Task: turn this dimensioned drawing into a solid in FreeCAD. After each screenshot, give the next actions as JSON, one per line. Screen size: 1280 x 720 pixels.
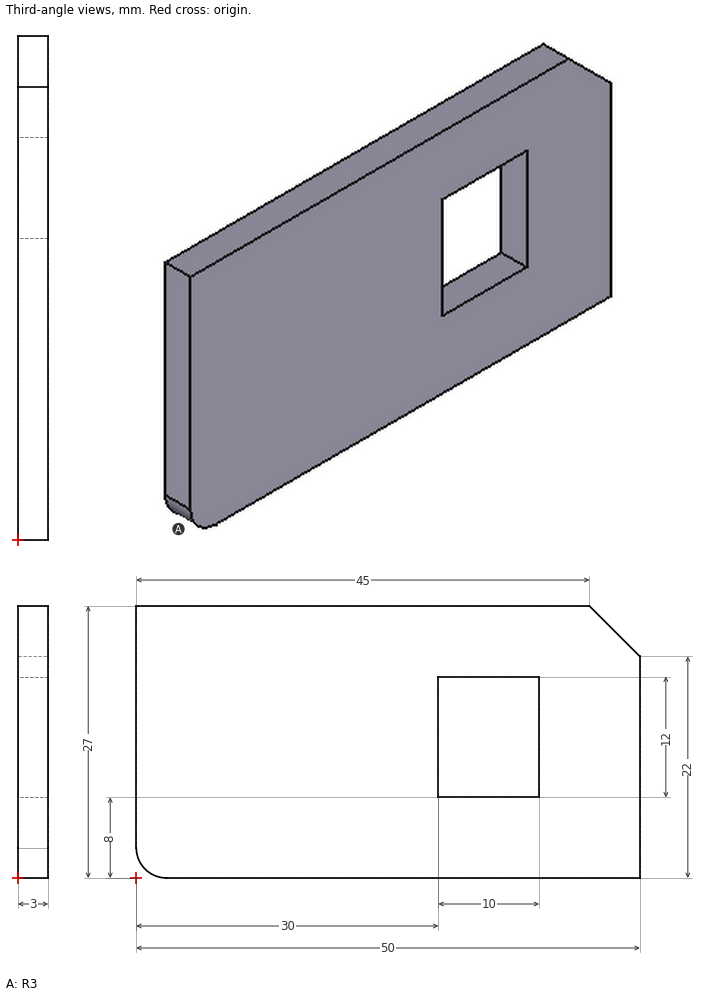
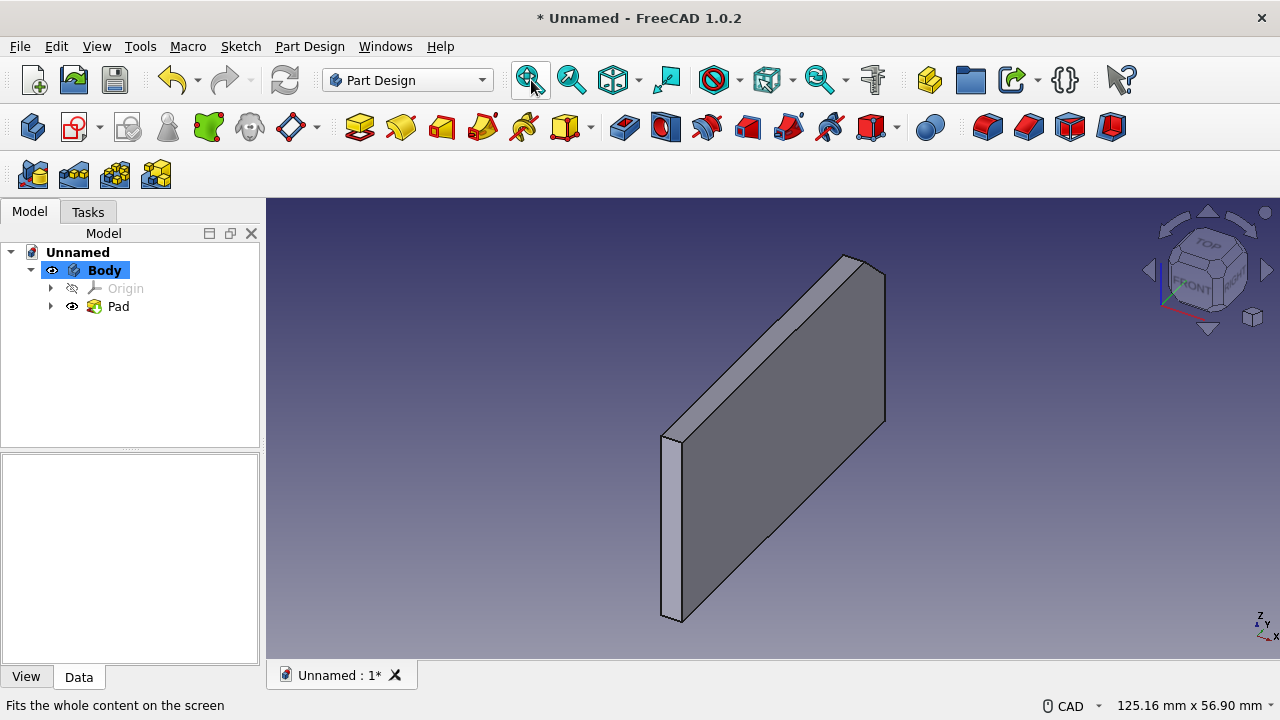
{"action": "key", "text": "0"}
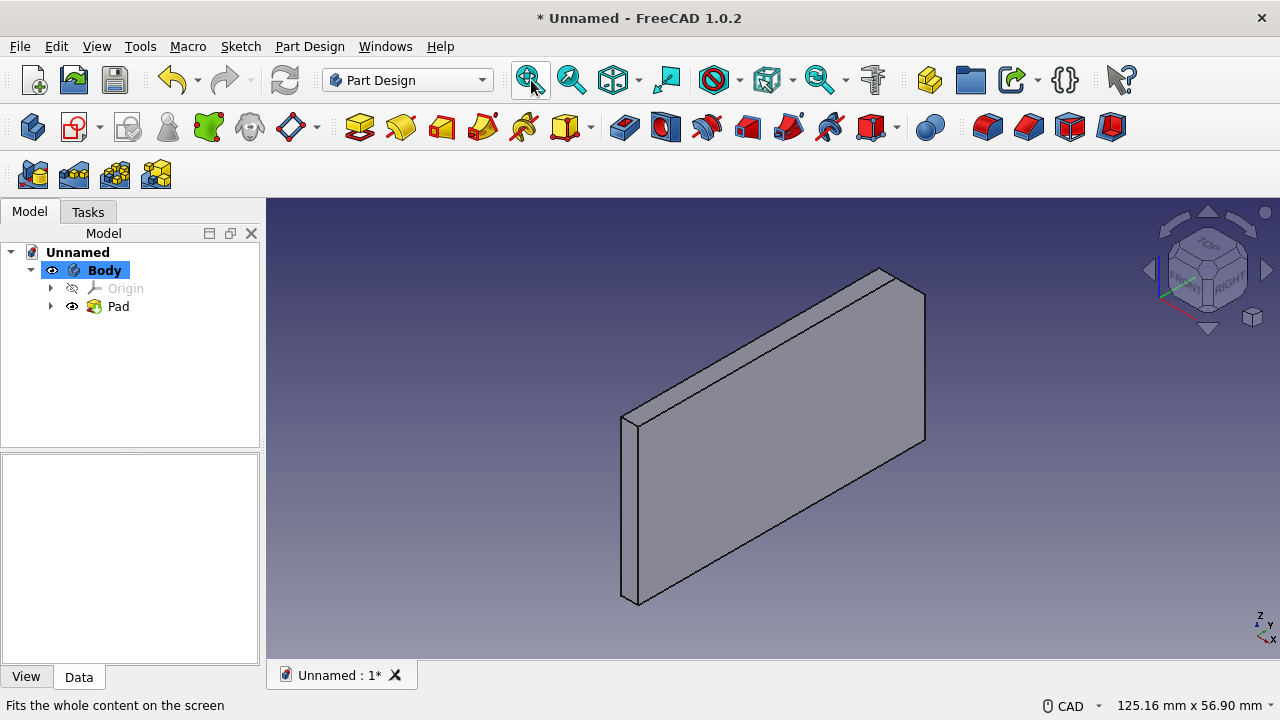
{"action": "key", "text": "2"}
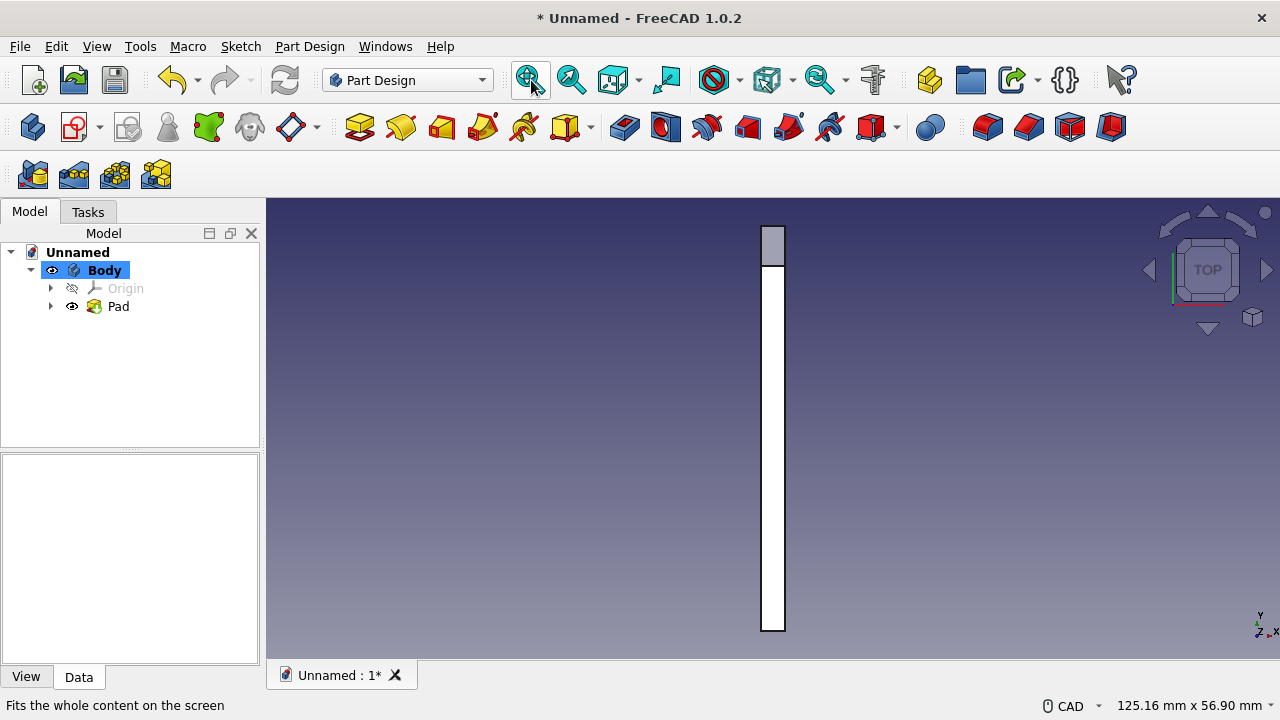
{"action": "key", "text": "1"}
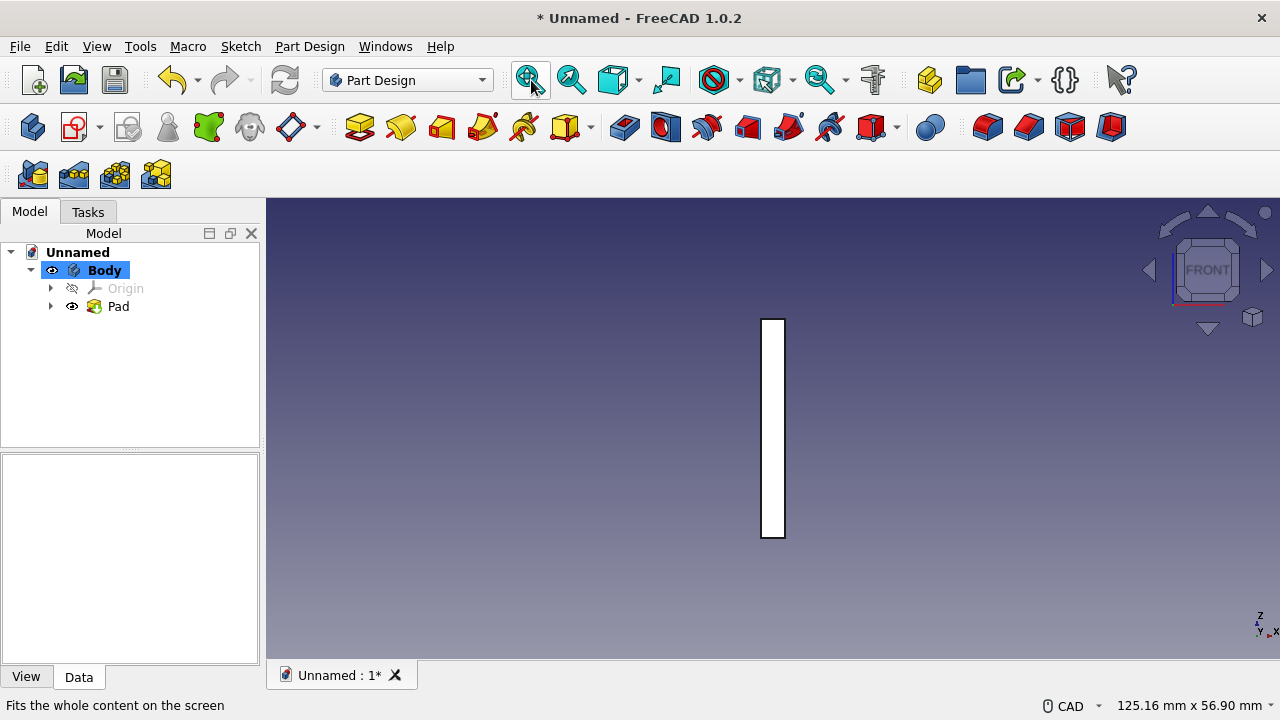
{"action": "key", "text": "3"}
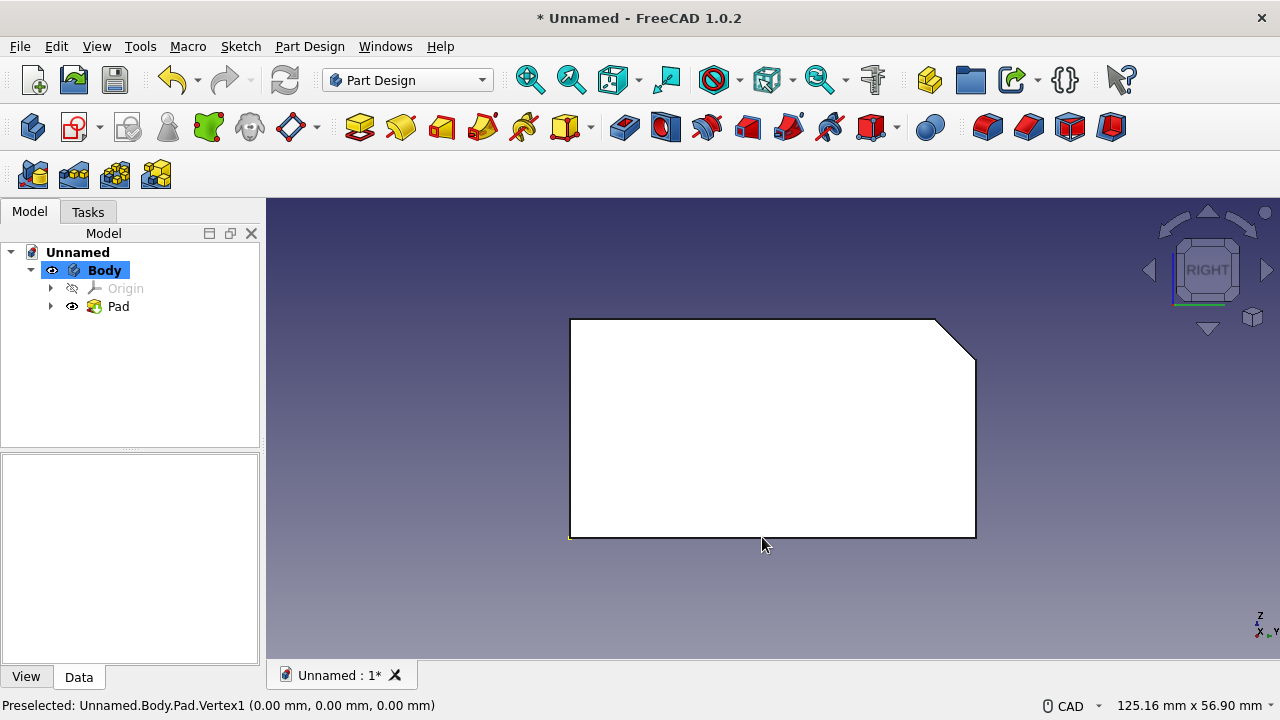
{"action": "key", "text": "5"}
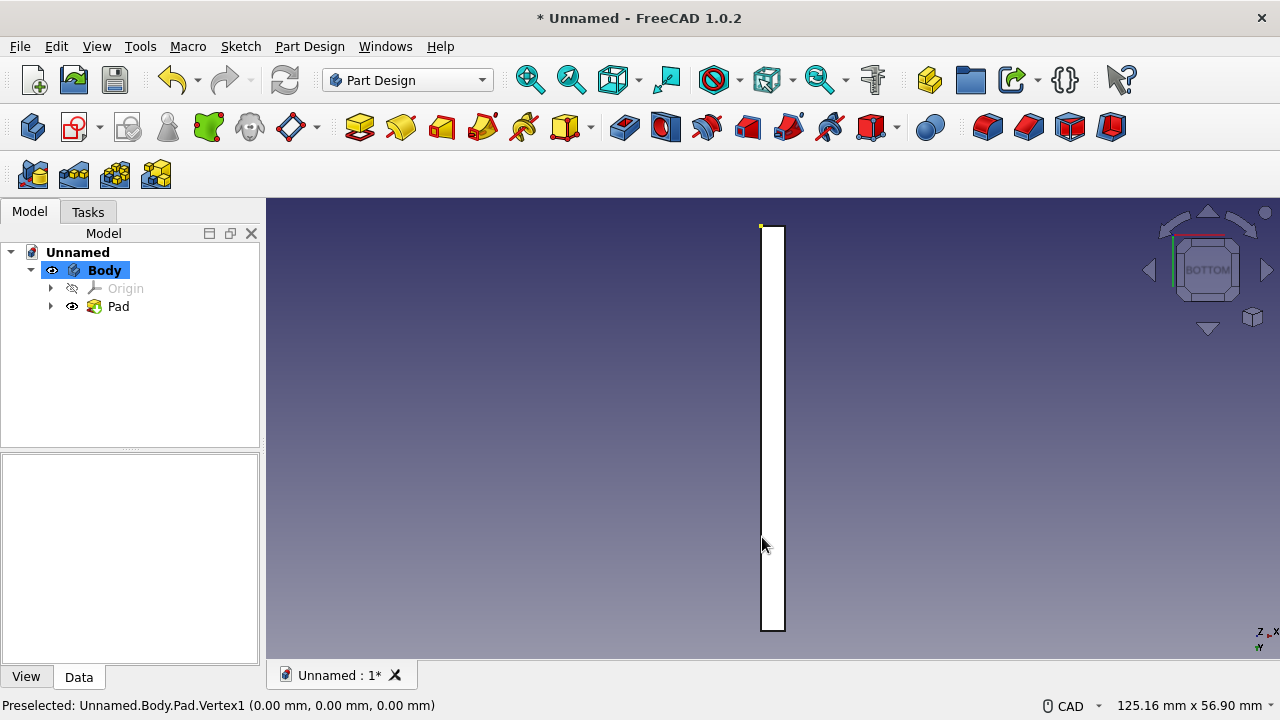
{"action": "key", "text": "4"}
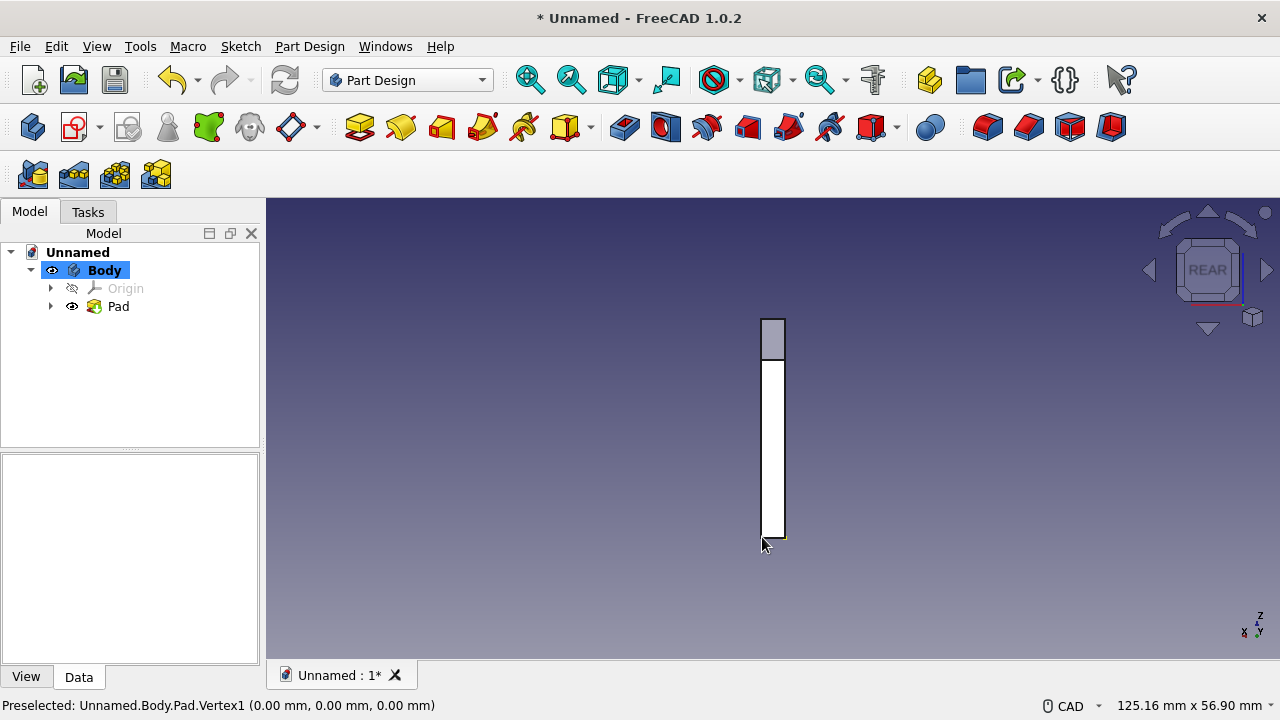
{"action": "key", "text": "6"}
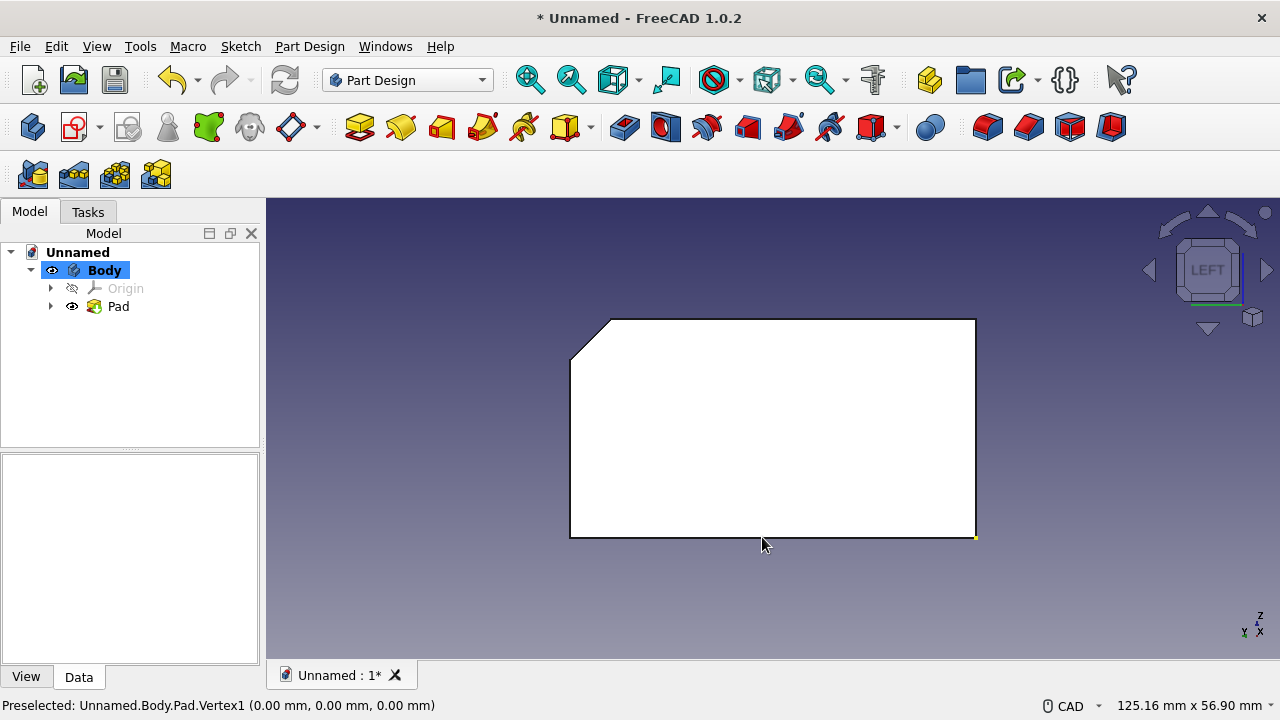
{"action": "key", "text": "v 3"}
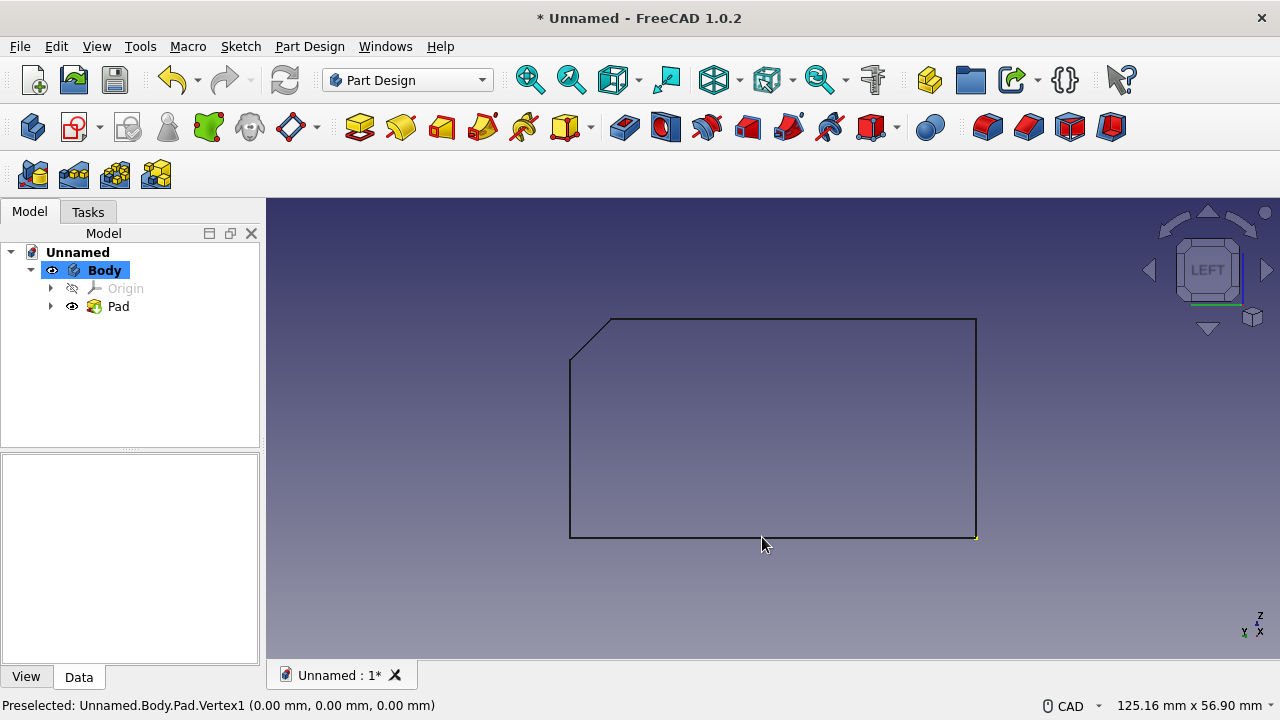
{"action": "key", "text": "0"}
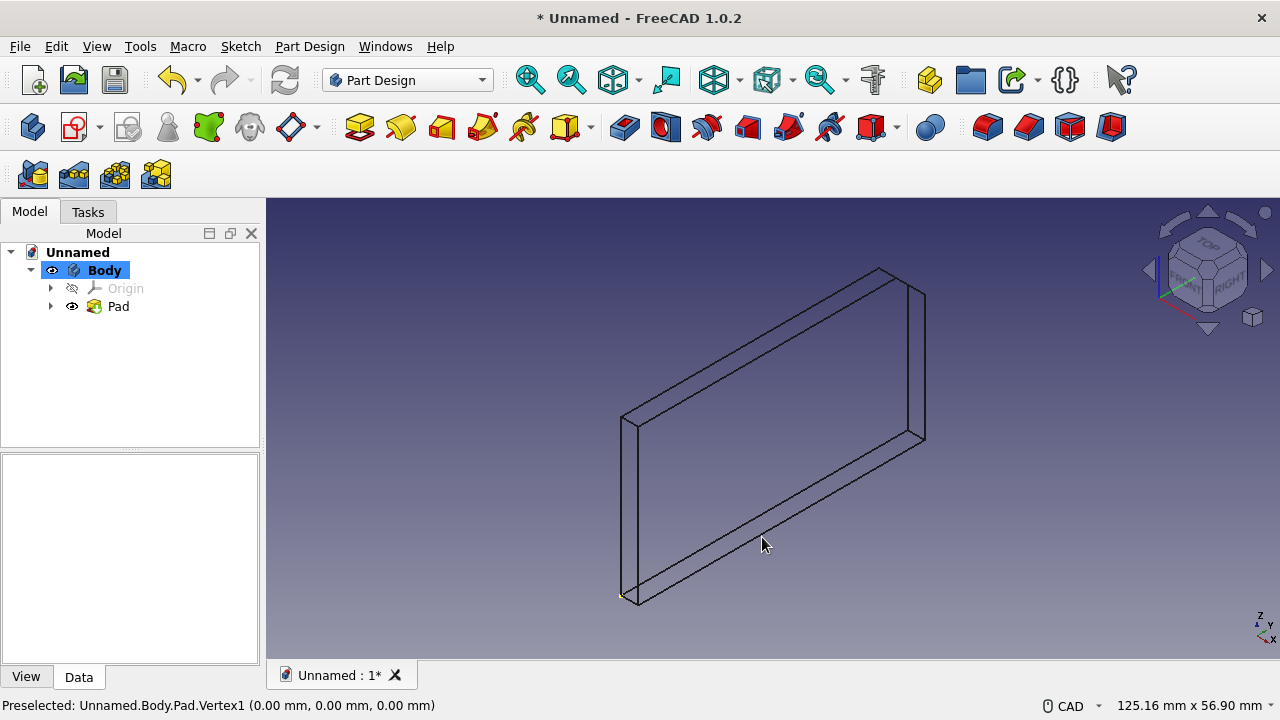
{"action": "left_click", "coordinate": [630, 599]}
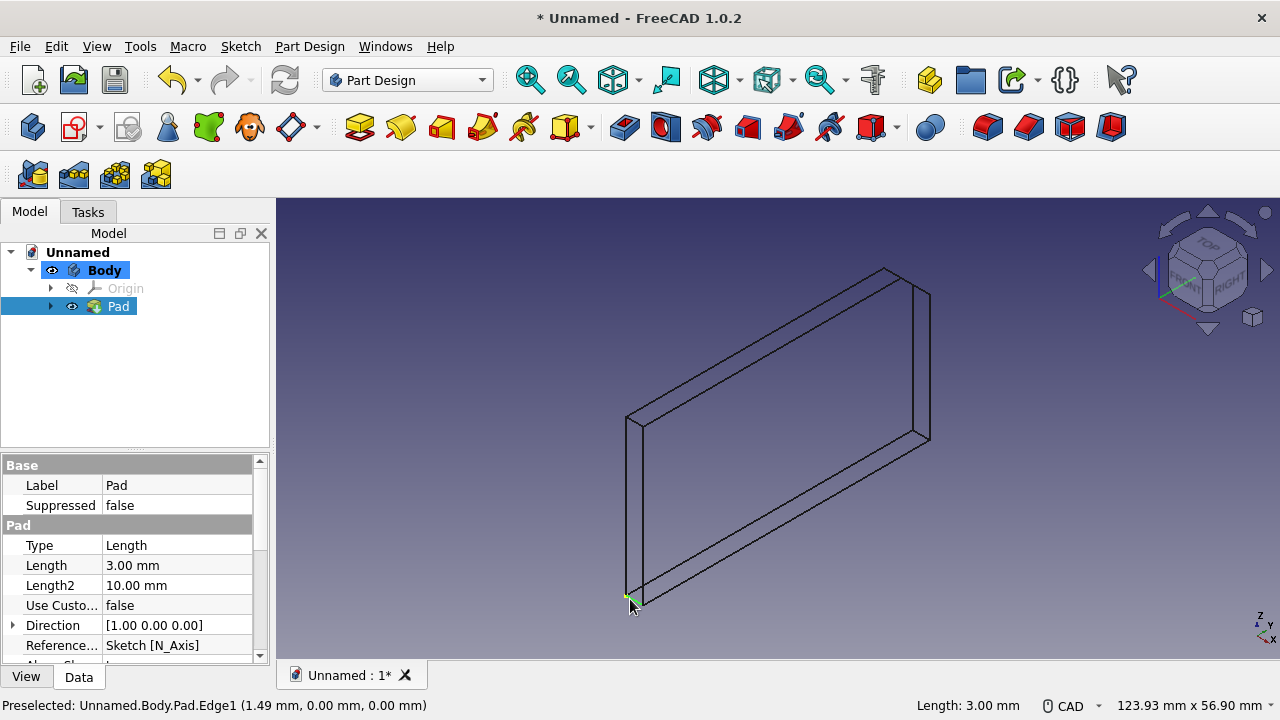
{"action": "key", "text": "v 1"}